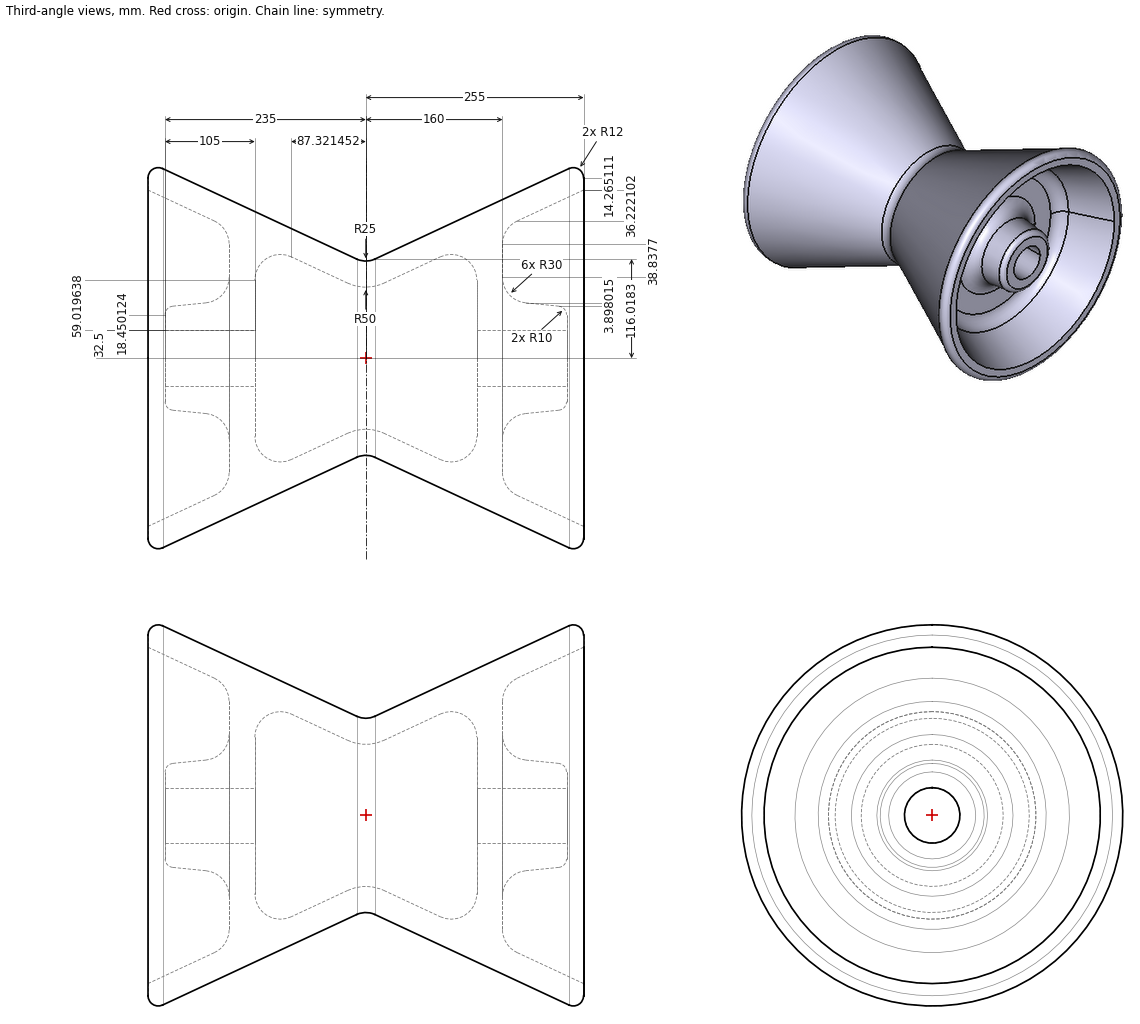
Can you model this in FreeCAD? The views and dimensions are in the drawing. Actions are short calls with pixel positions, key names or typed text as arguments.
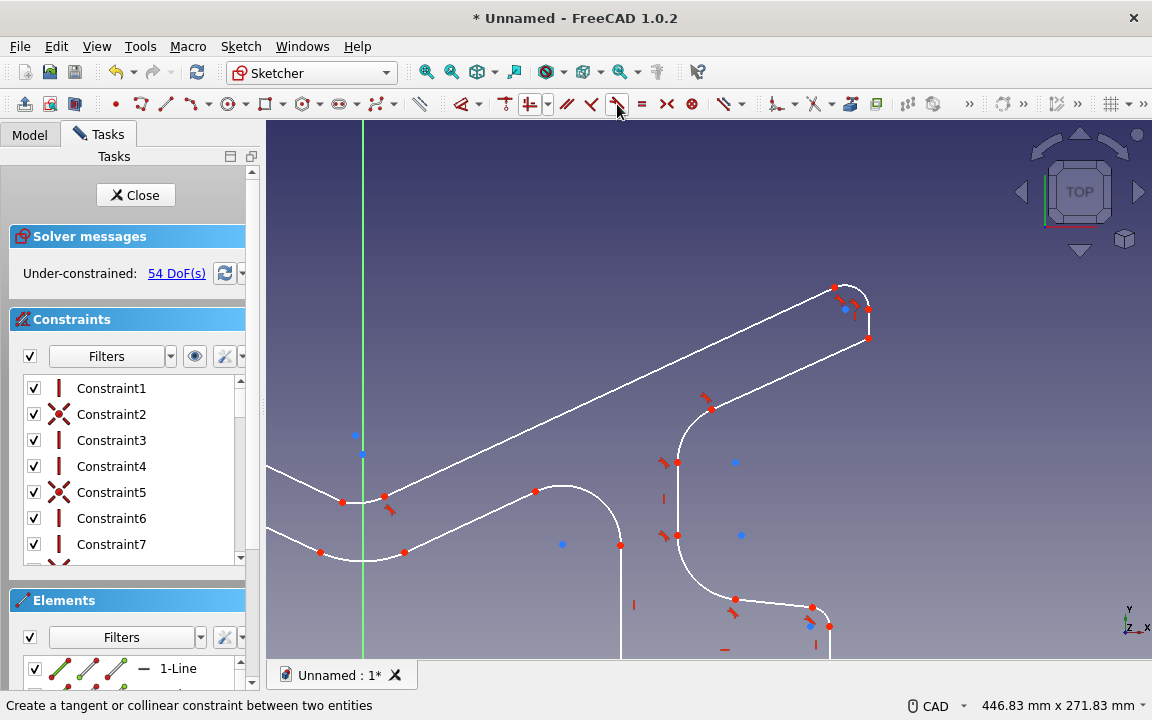
scroll(867, 295, down, 4)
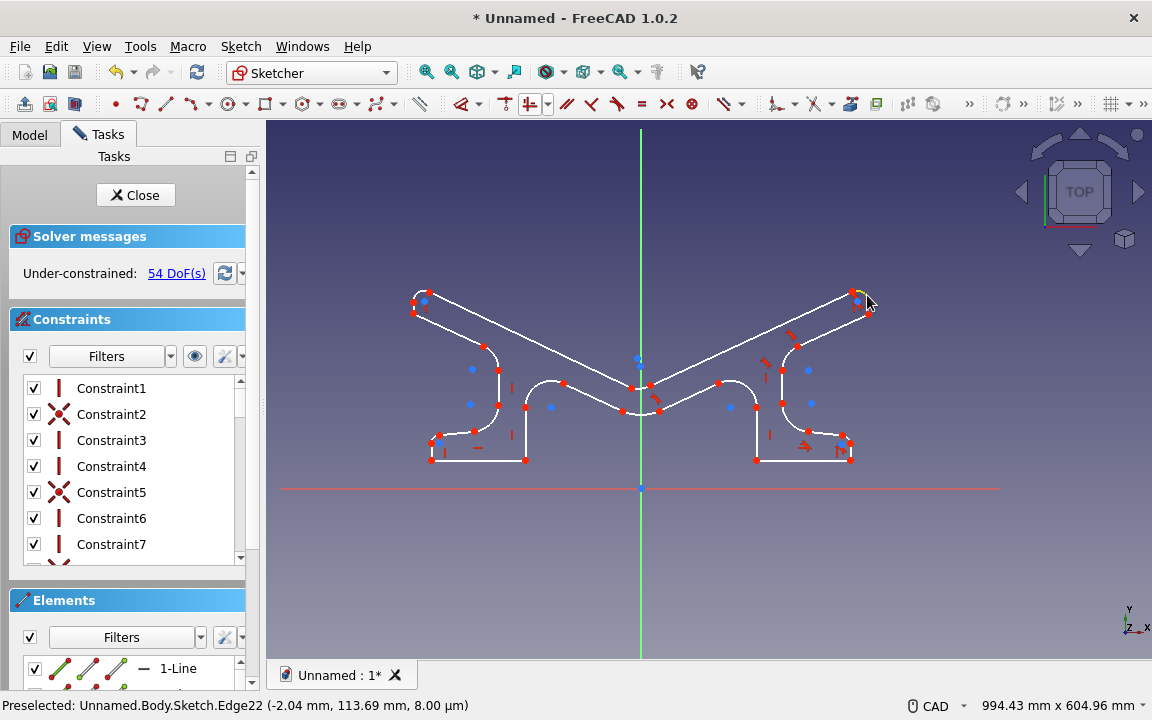
click(571, 359)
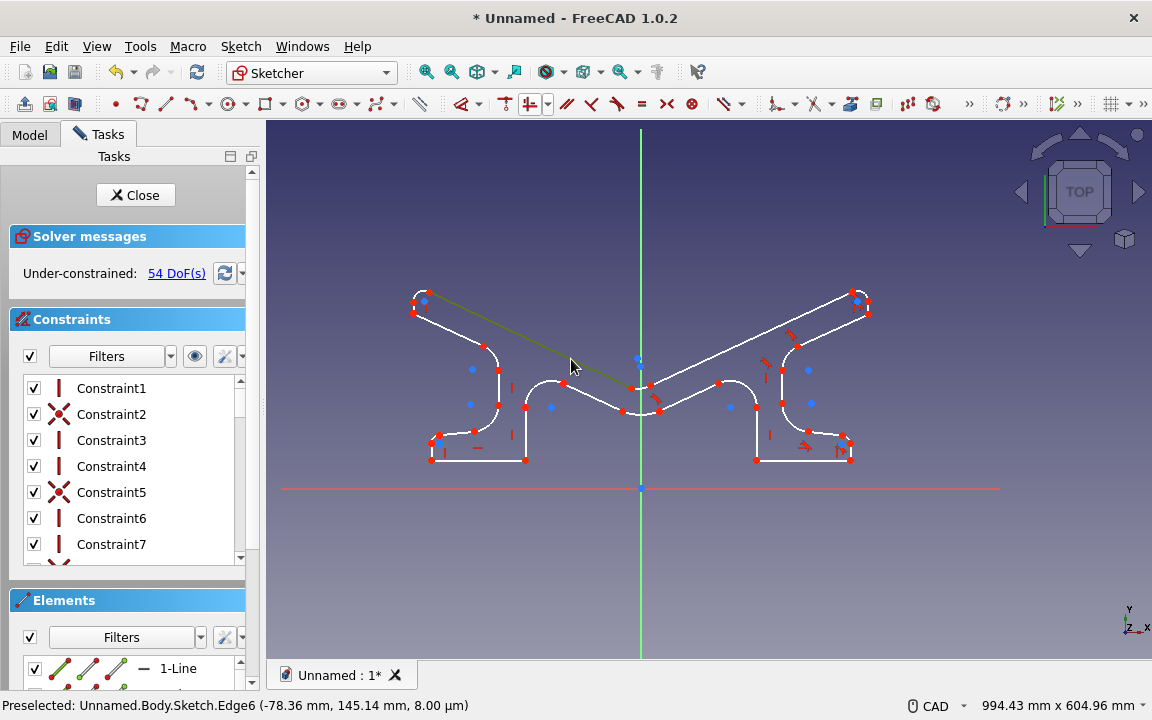
scroll(641, 389, up, 2)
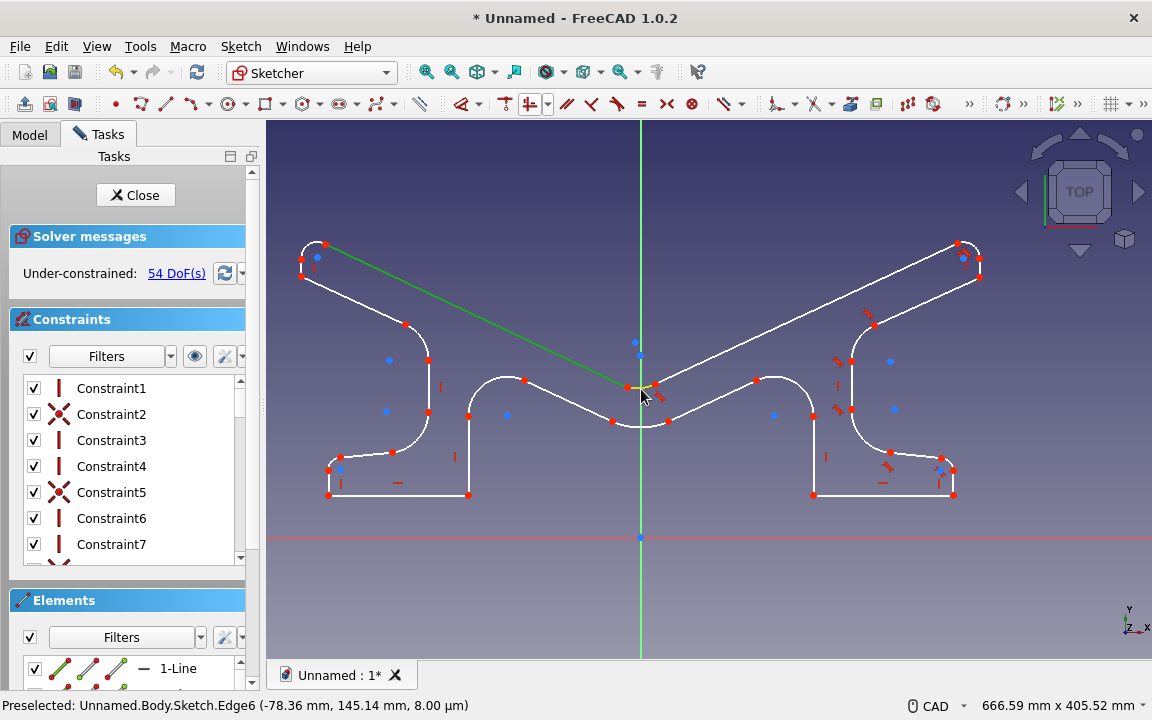
click(641, 388)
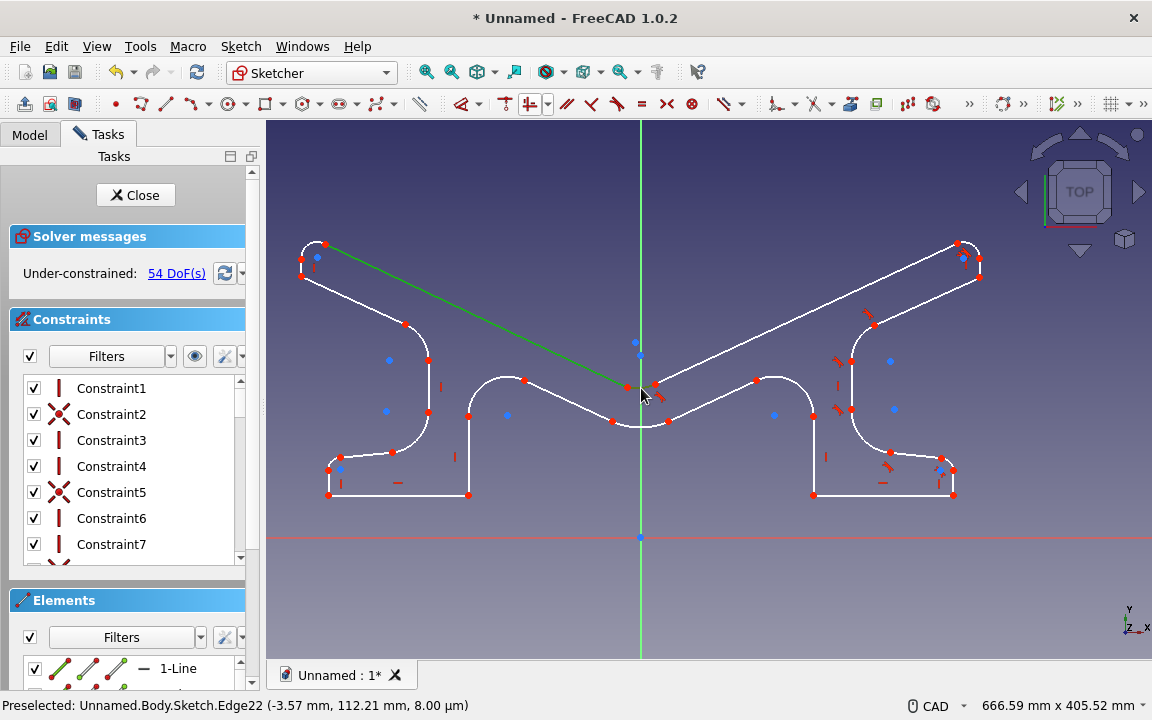
click(617, 104)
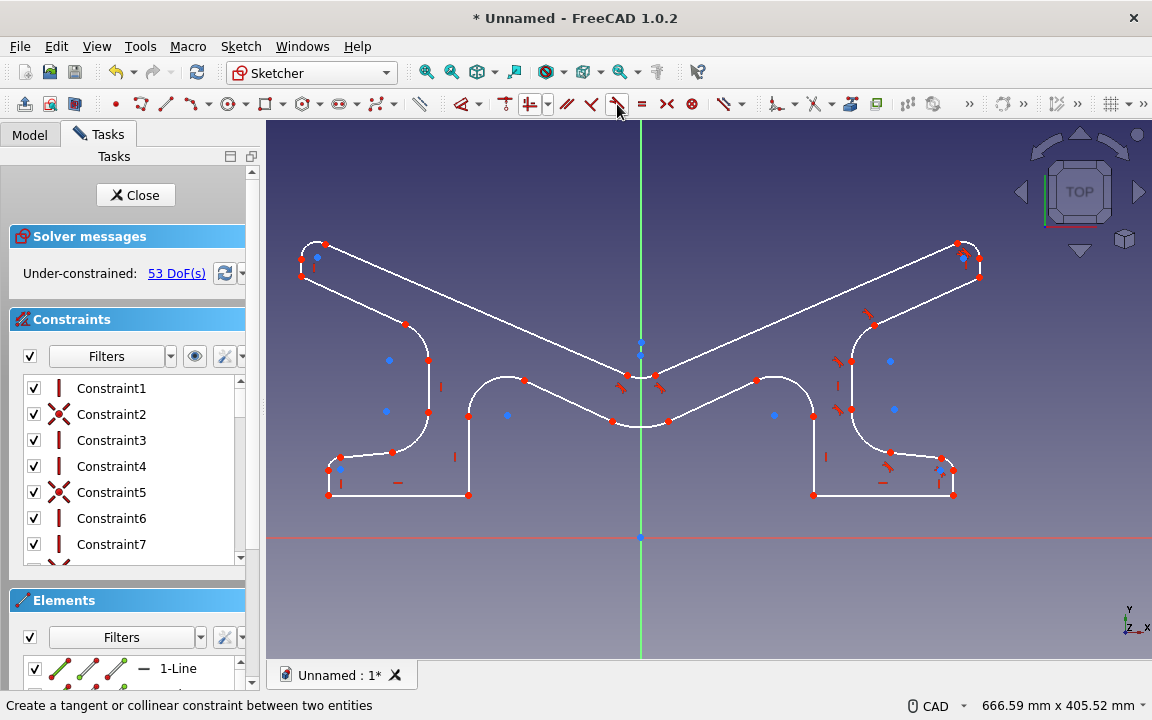
click(537, 336)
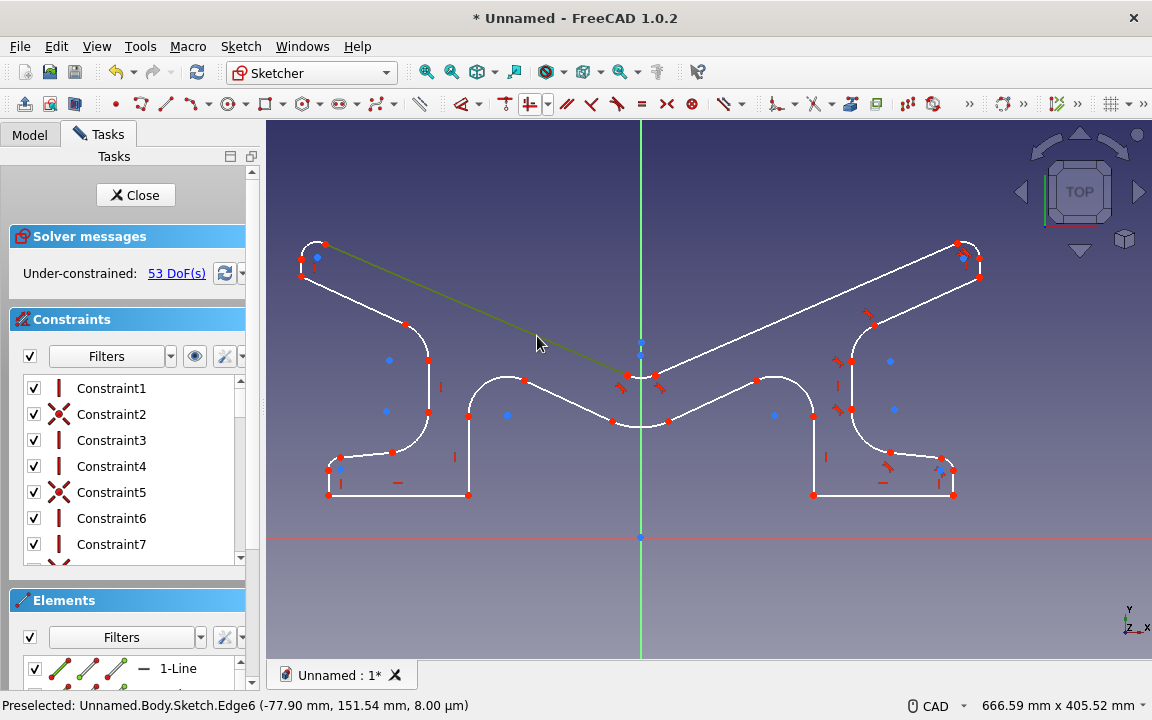
scroll(315, 242, up, 2)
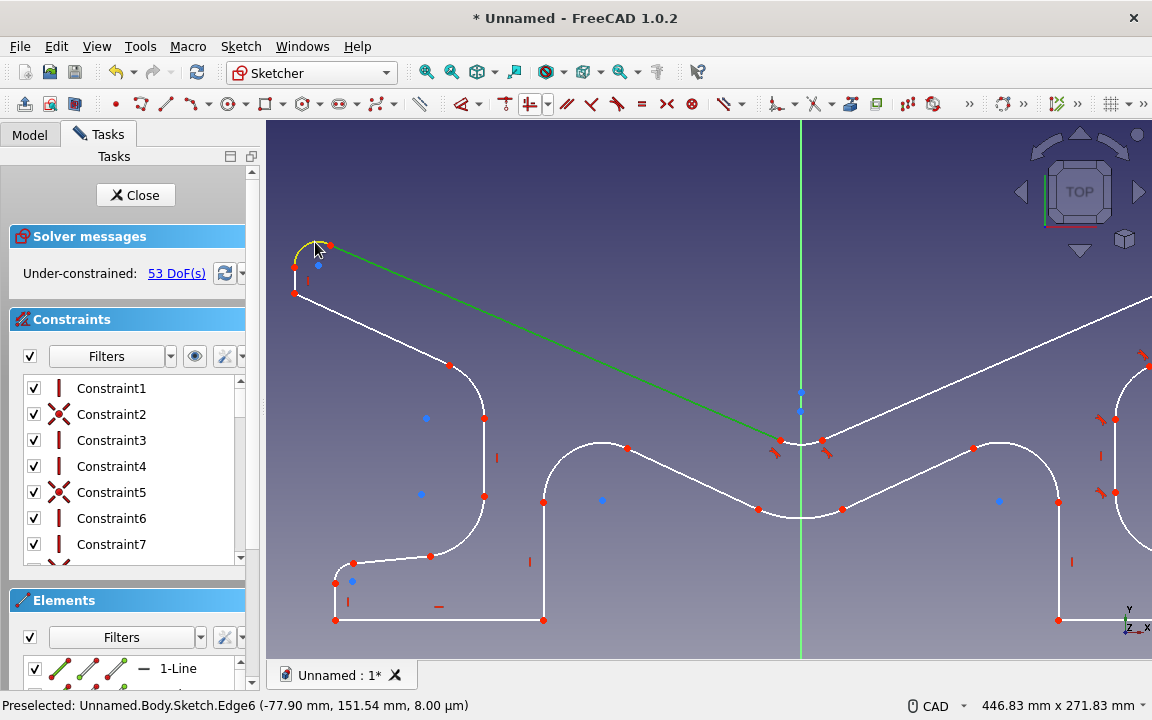
click(315, 242)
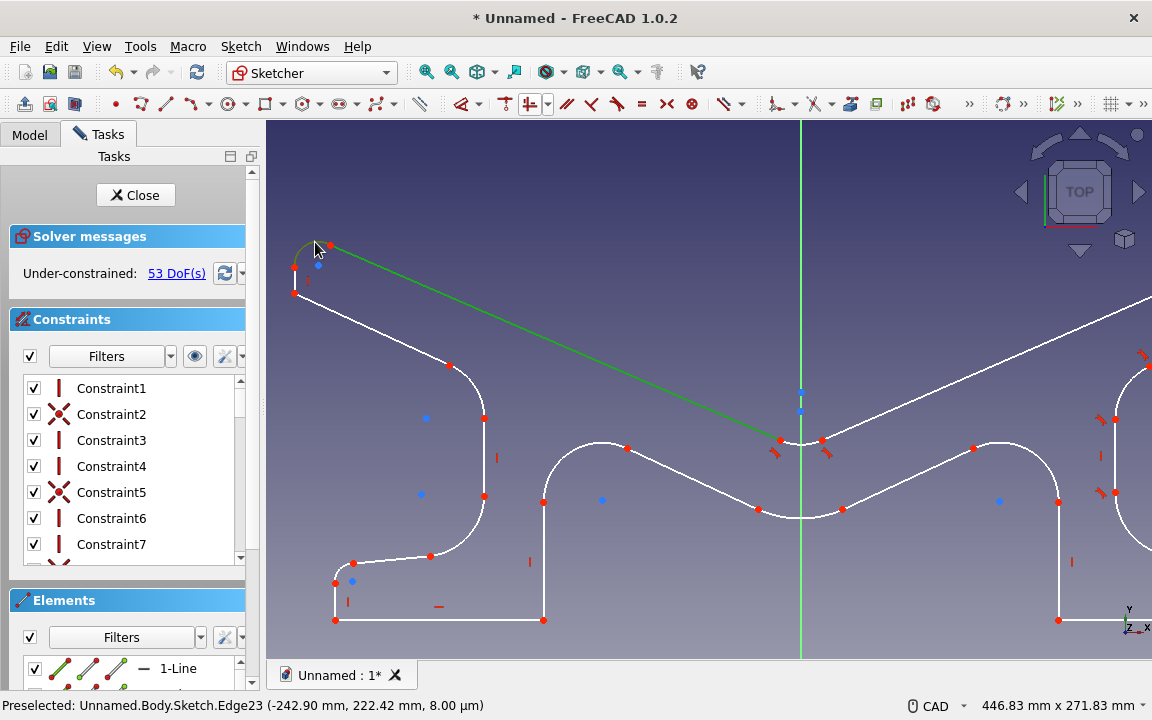
click(617, 104)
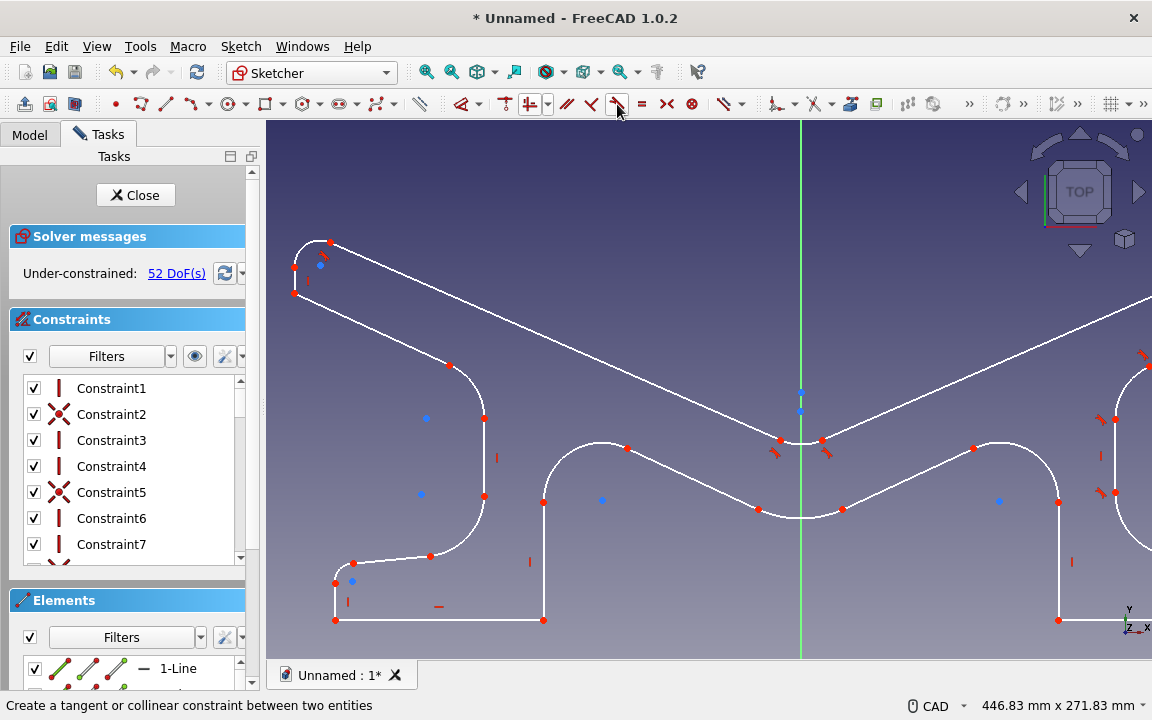
scroll(295, 278, up, 2)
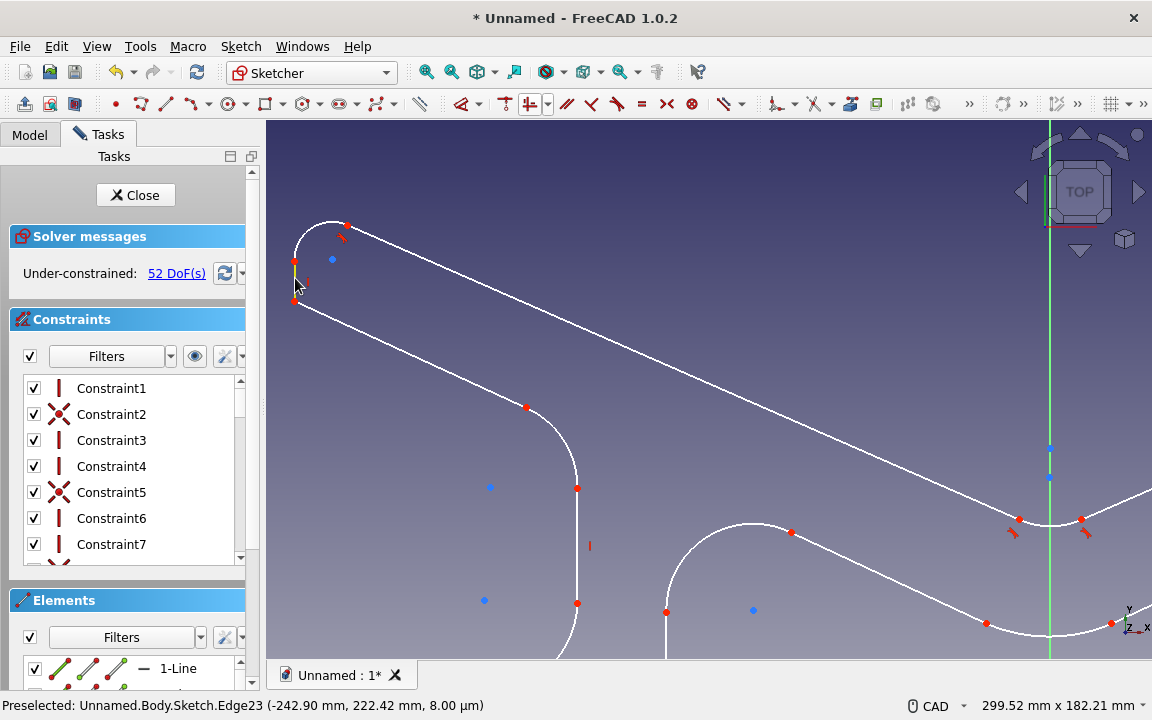
click(295, 278)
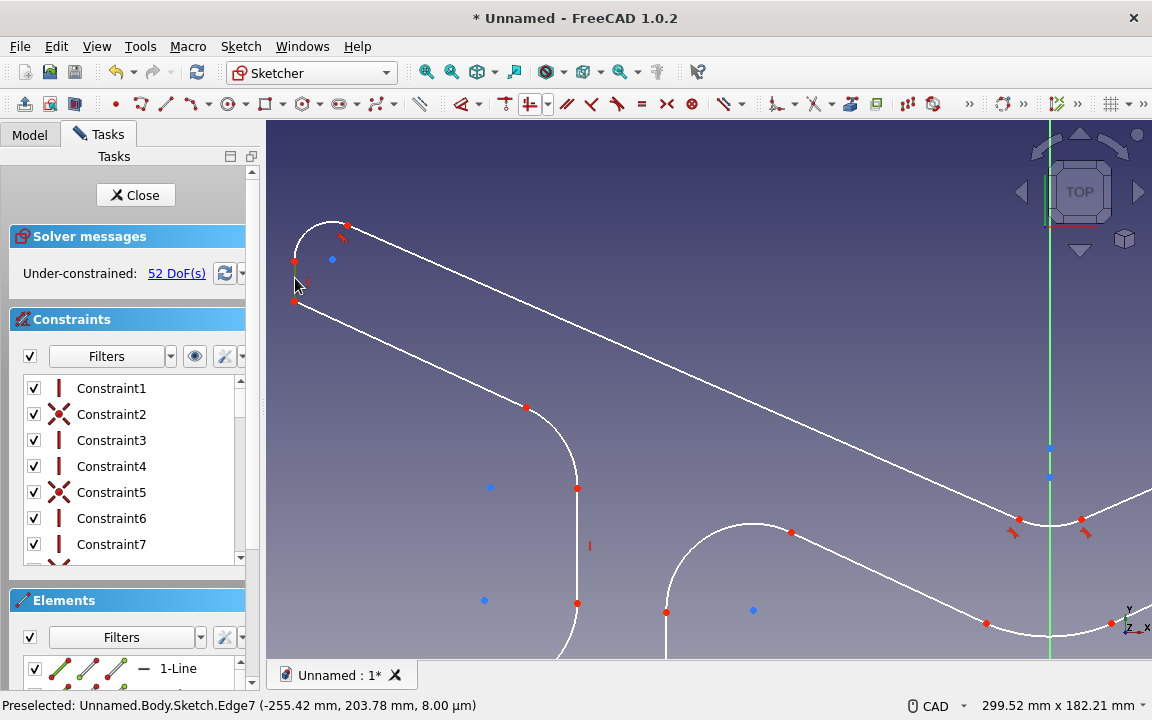
click(325, 223)